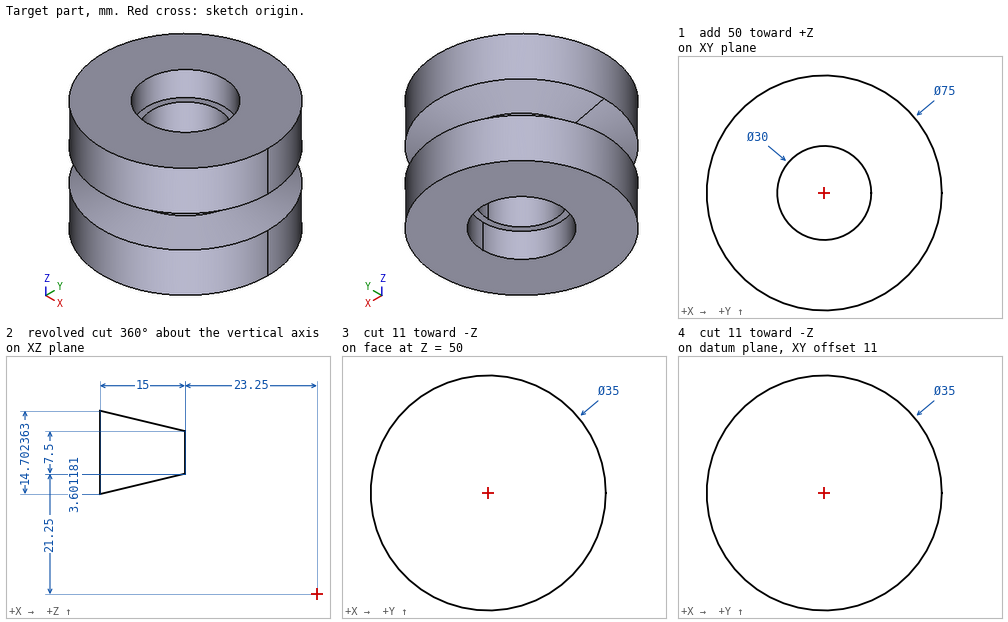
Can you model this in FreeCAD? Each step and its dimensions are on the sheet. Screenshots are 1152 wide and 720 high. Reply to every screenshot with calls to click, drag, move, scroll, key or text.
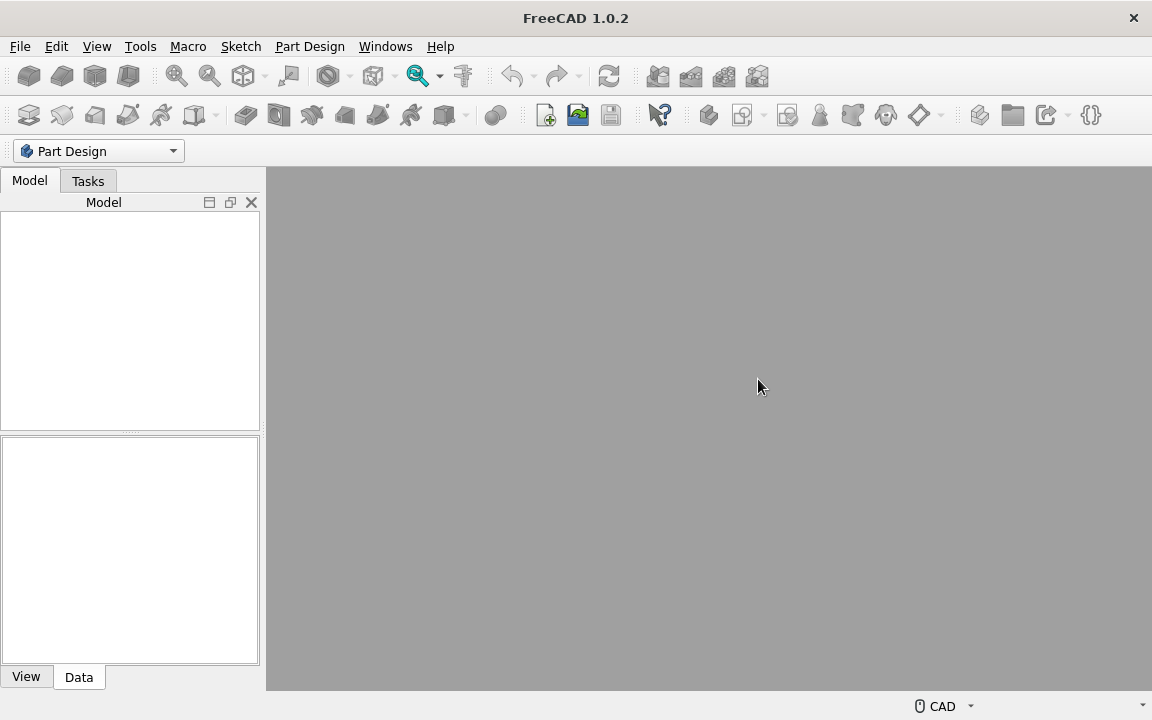
click(545, 116)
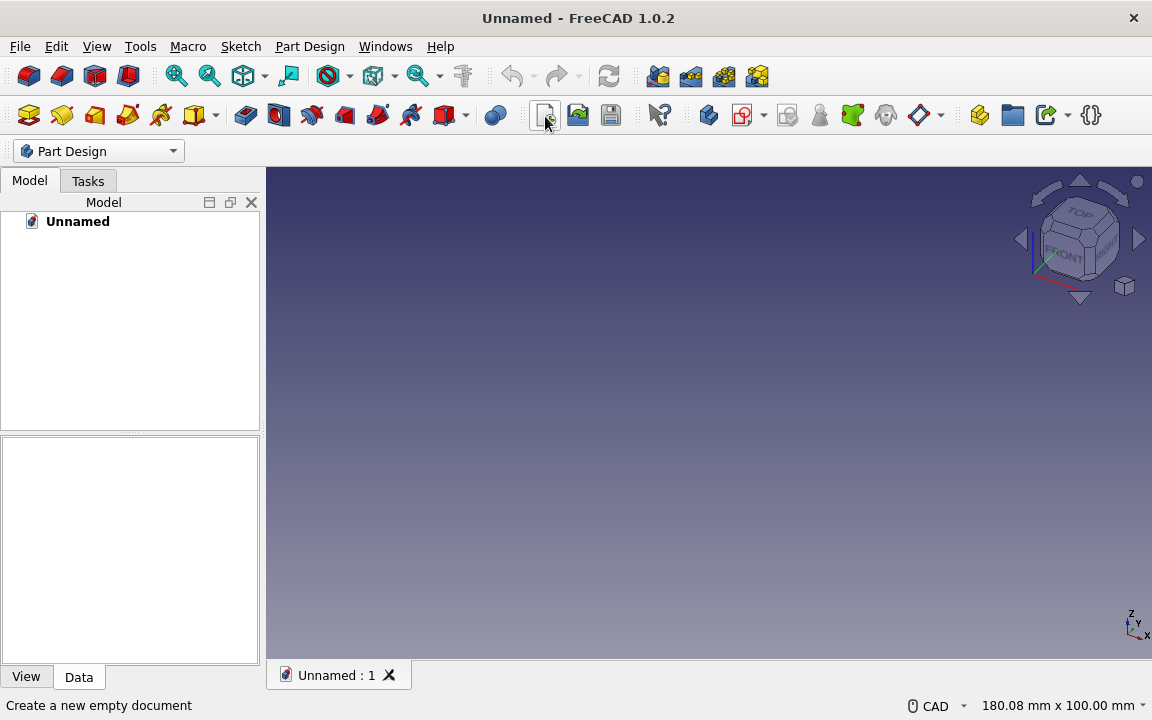
click(742, 116)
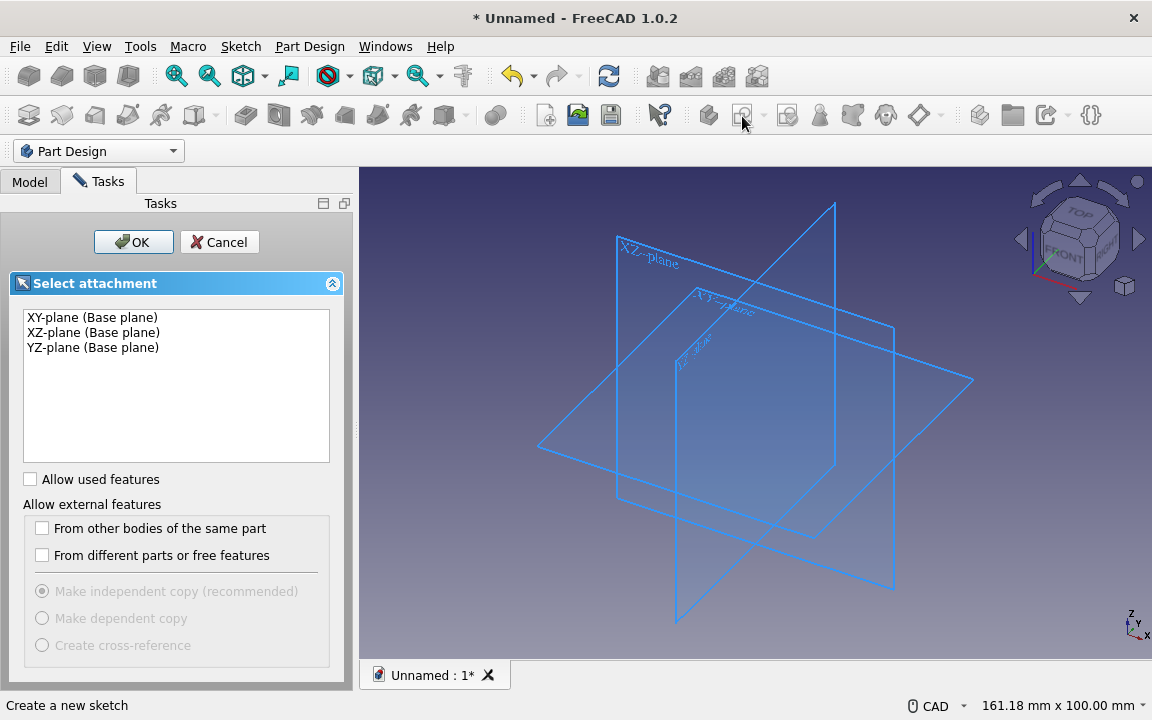
click(84, 318)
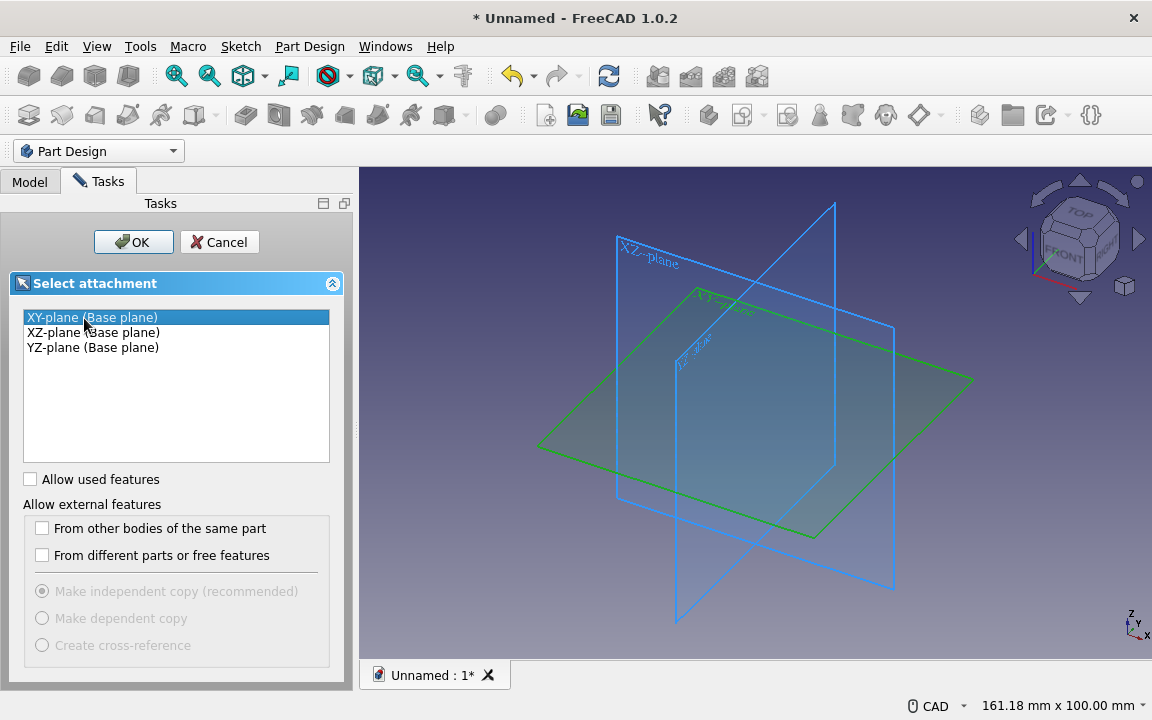
click(134, 242)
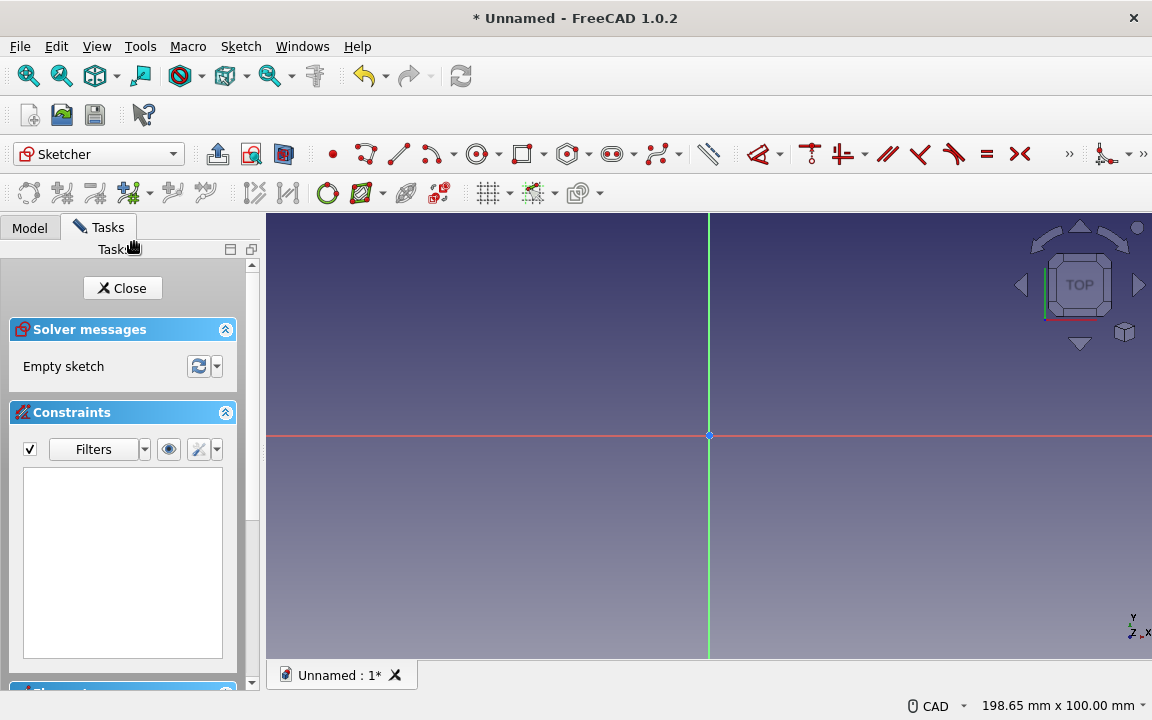
key(g)
key(c)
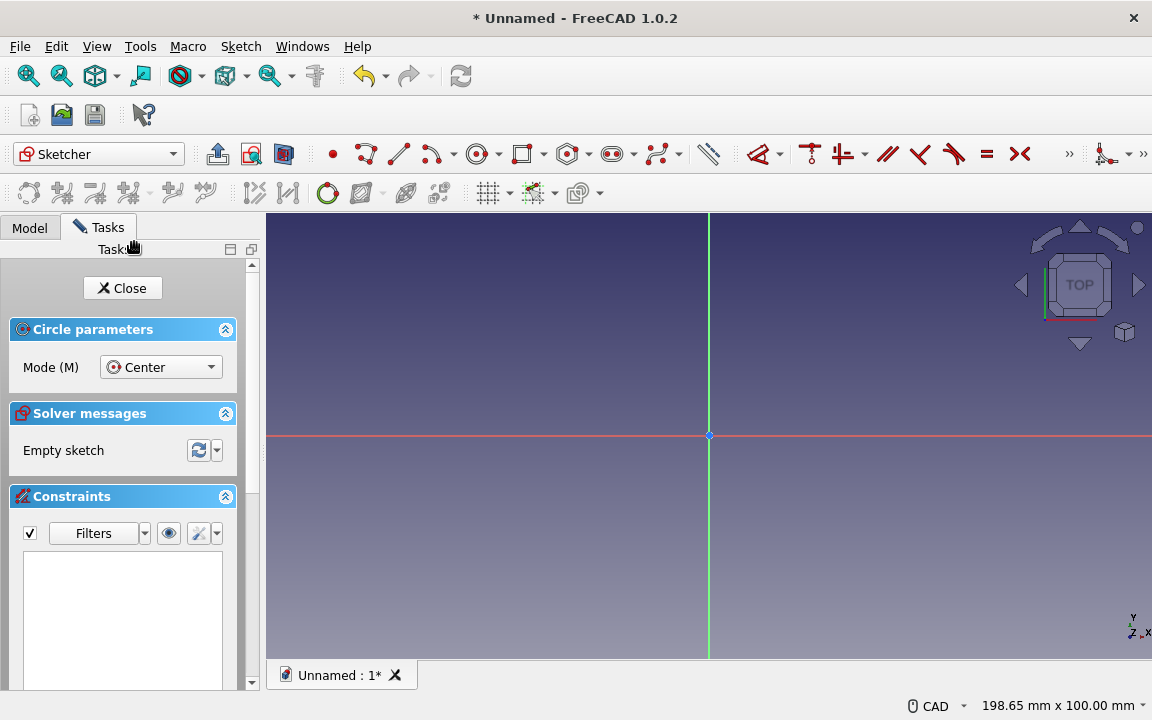
click(709, 436)
move(827, 318)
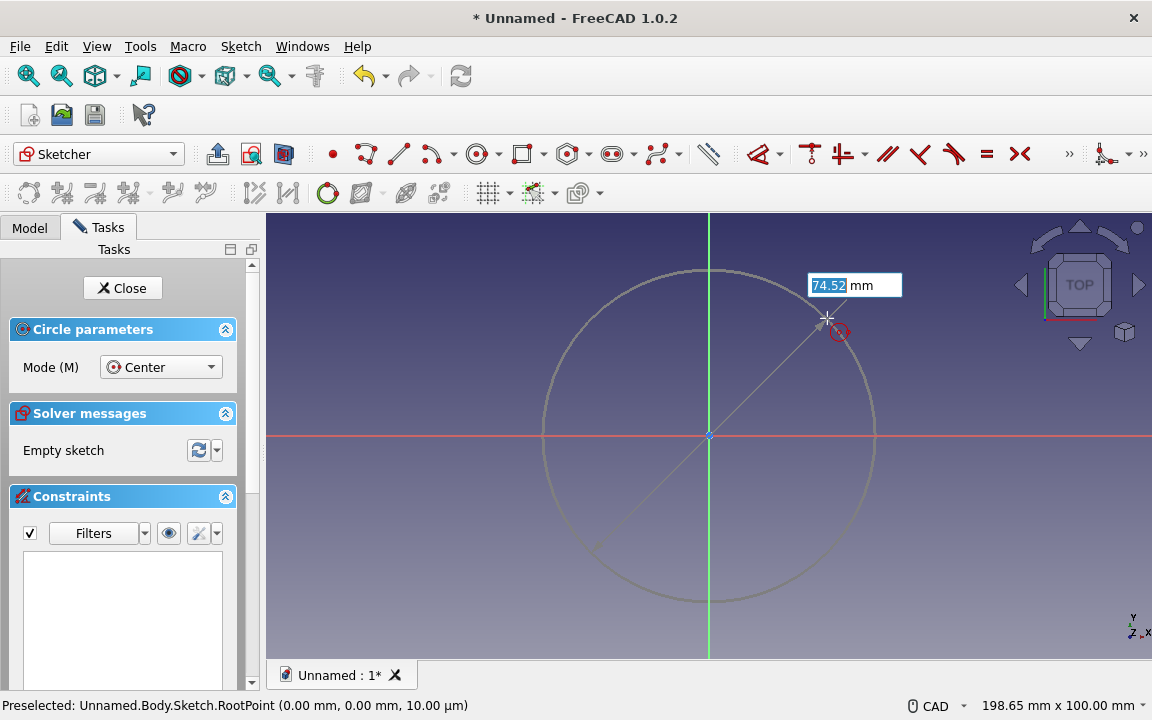
text(75)
key(Return)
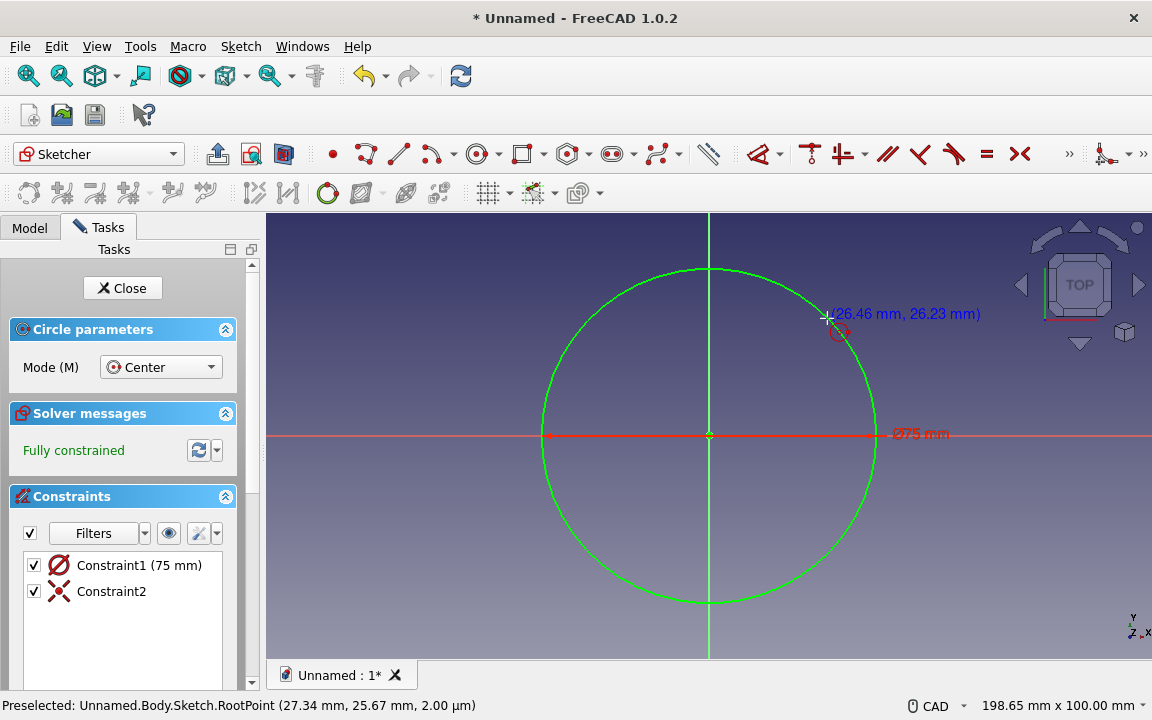
click(709, 436)
move(756, 389)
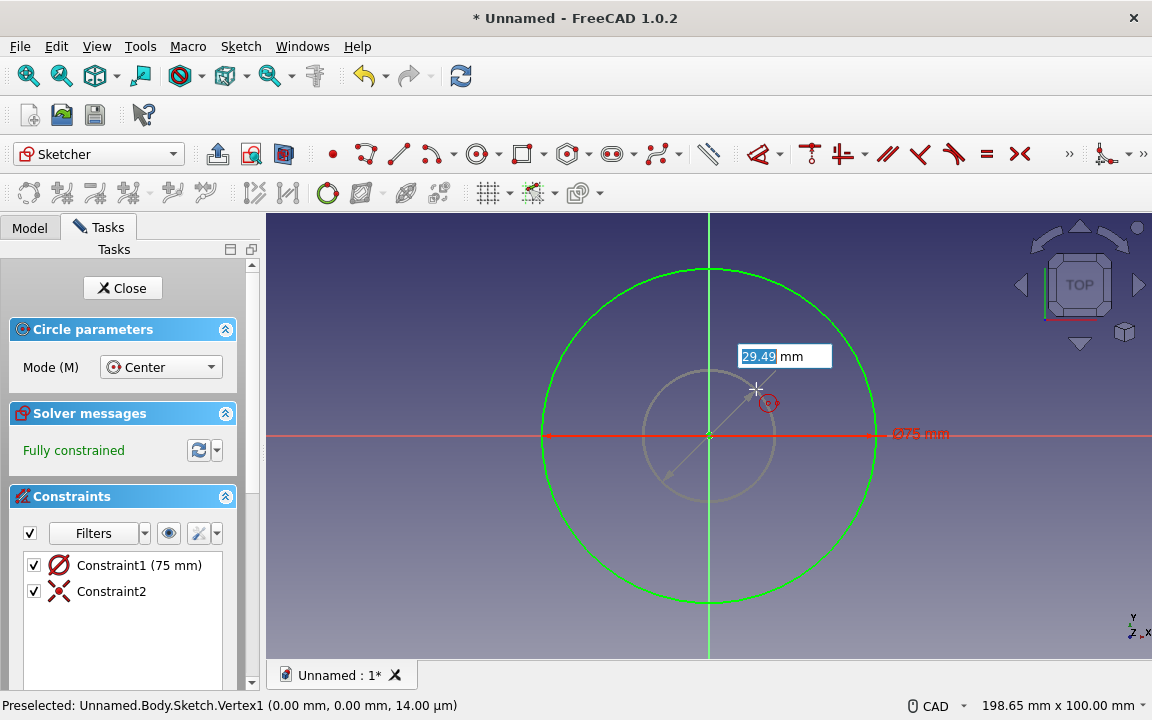
text(30)
key(Return)
key(Escape)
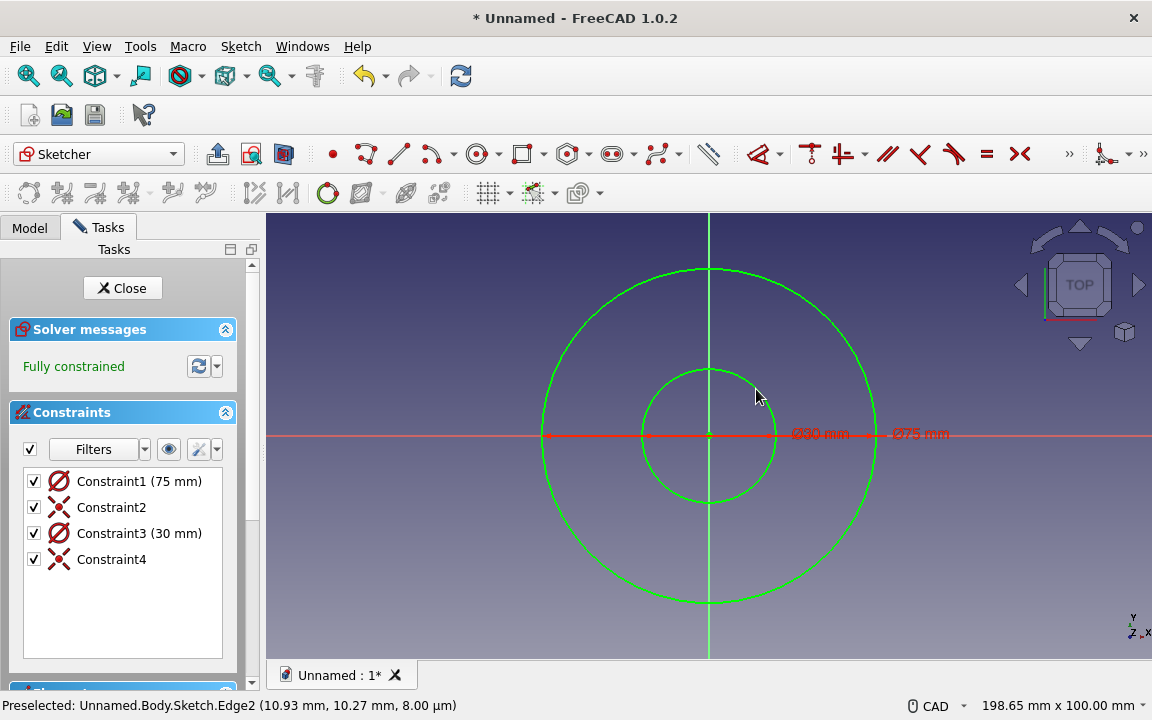
click(123, 288)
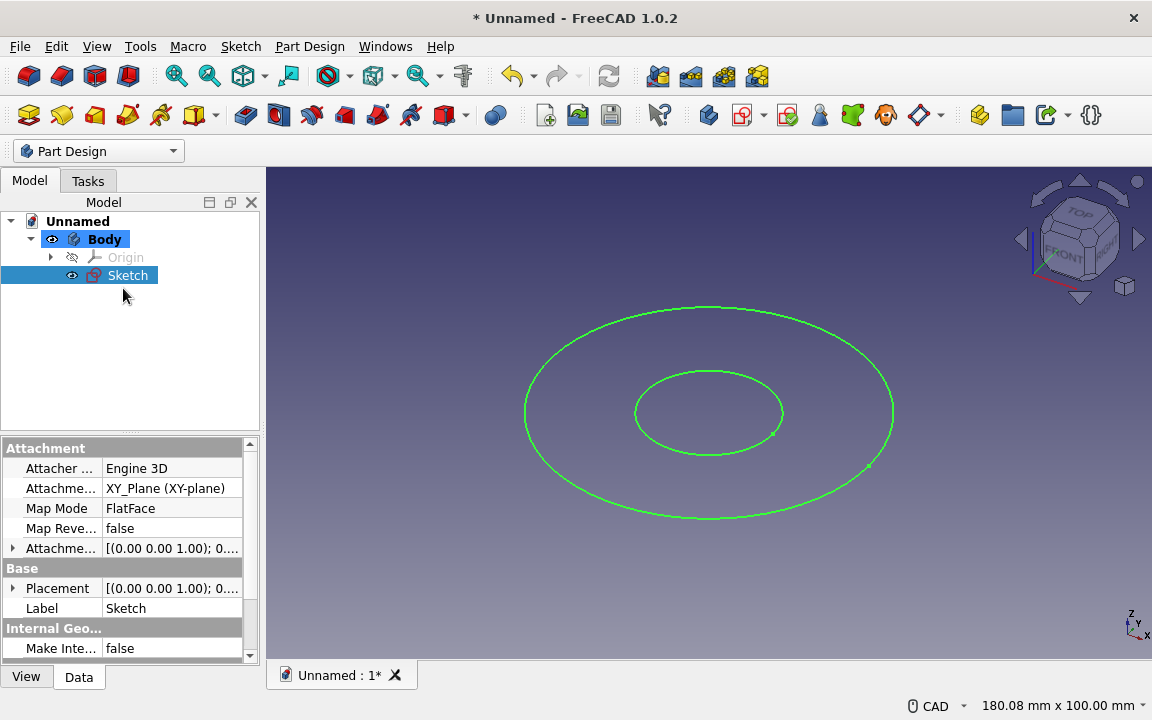
click(29, 116)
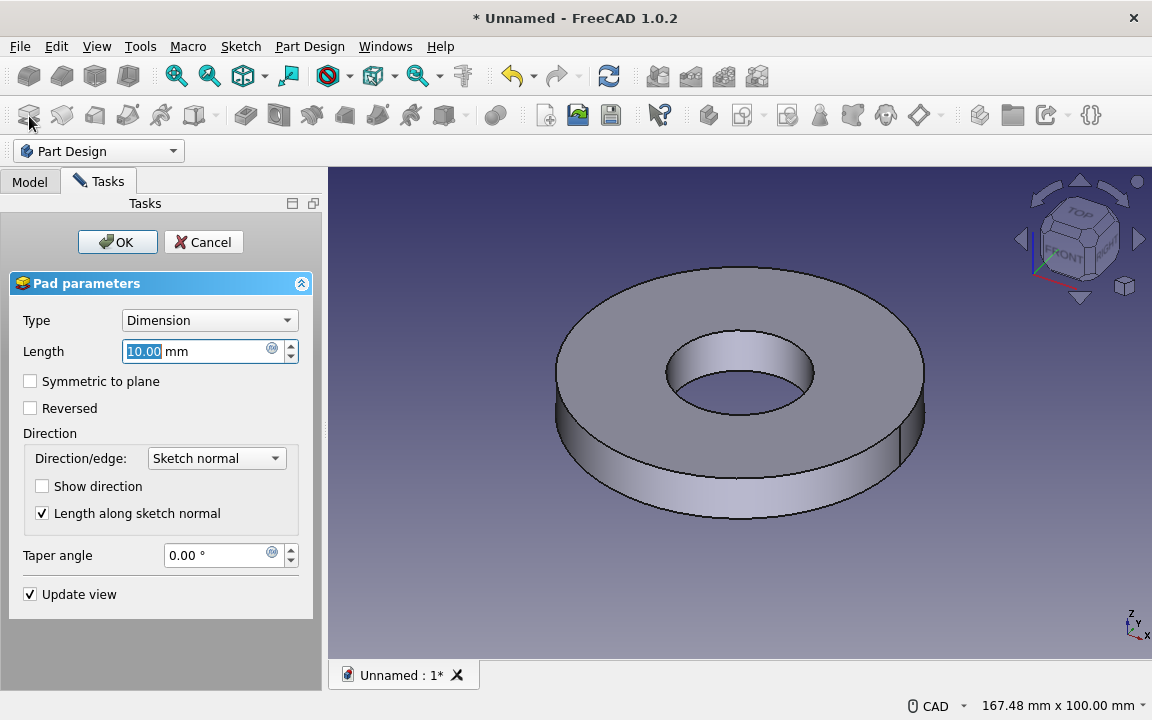
text(50)
key(Tab)